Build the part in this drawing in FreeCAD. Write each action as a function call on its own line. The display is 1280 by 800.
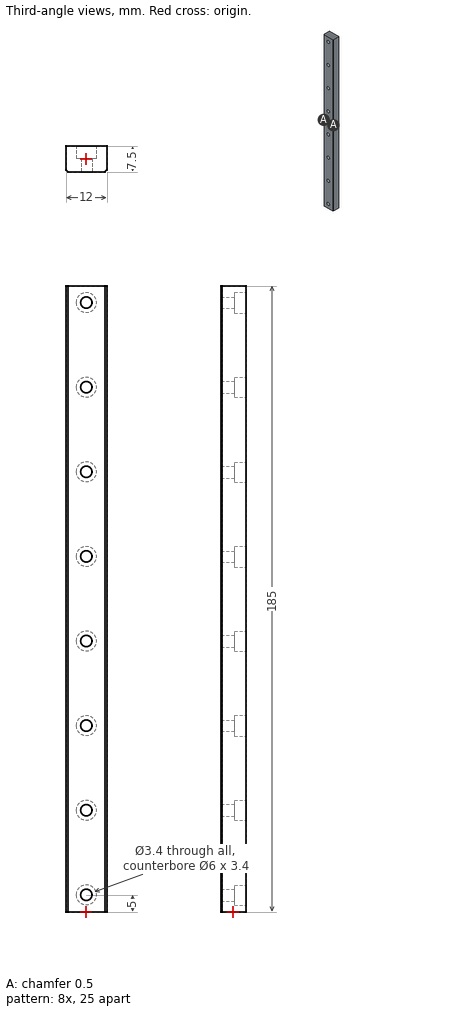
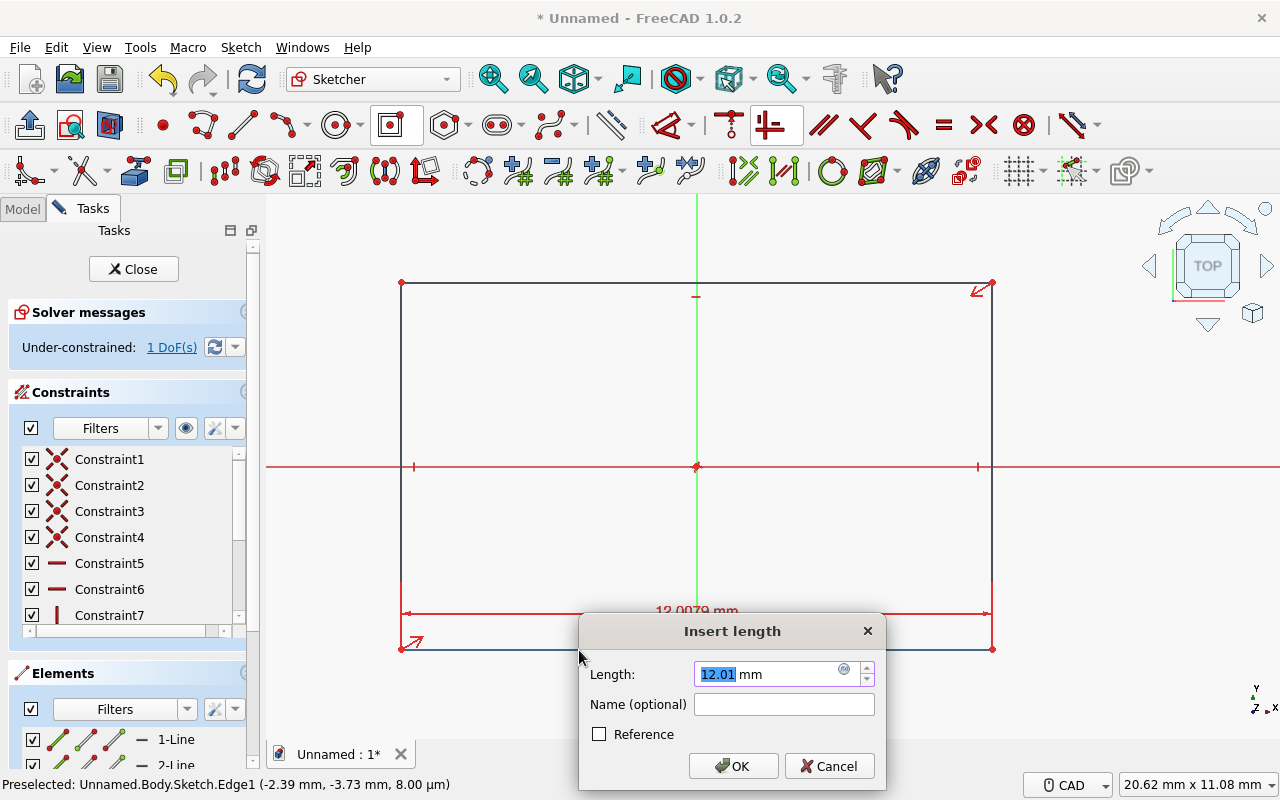
text(12)
key(Return)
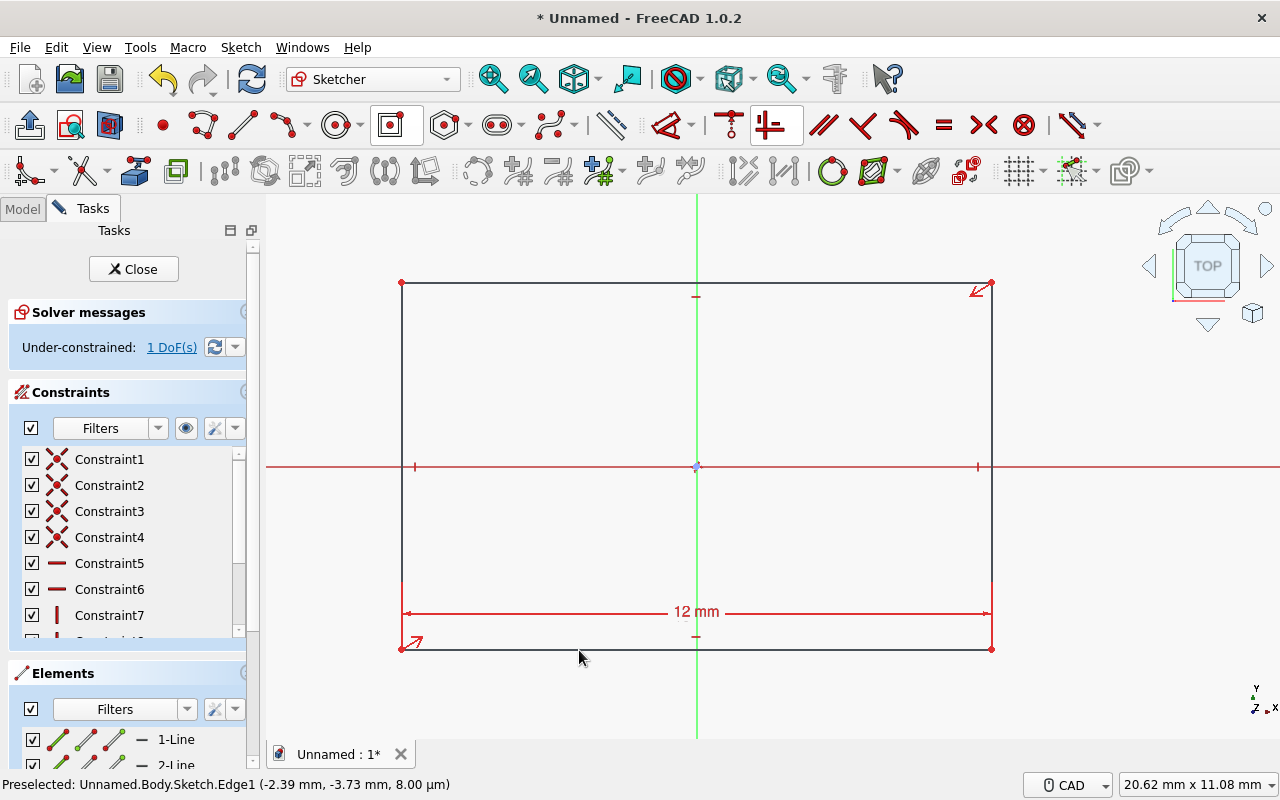
click(992, 540)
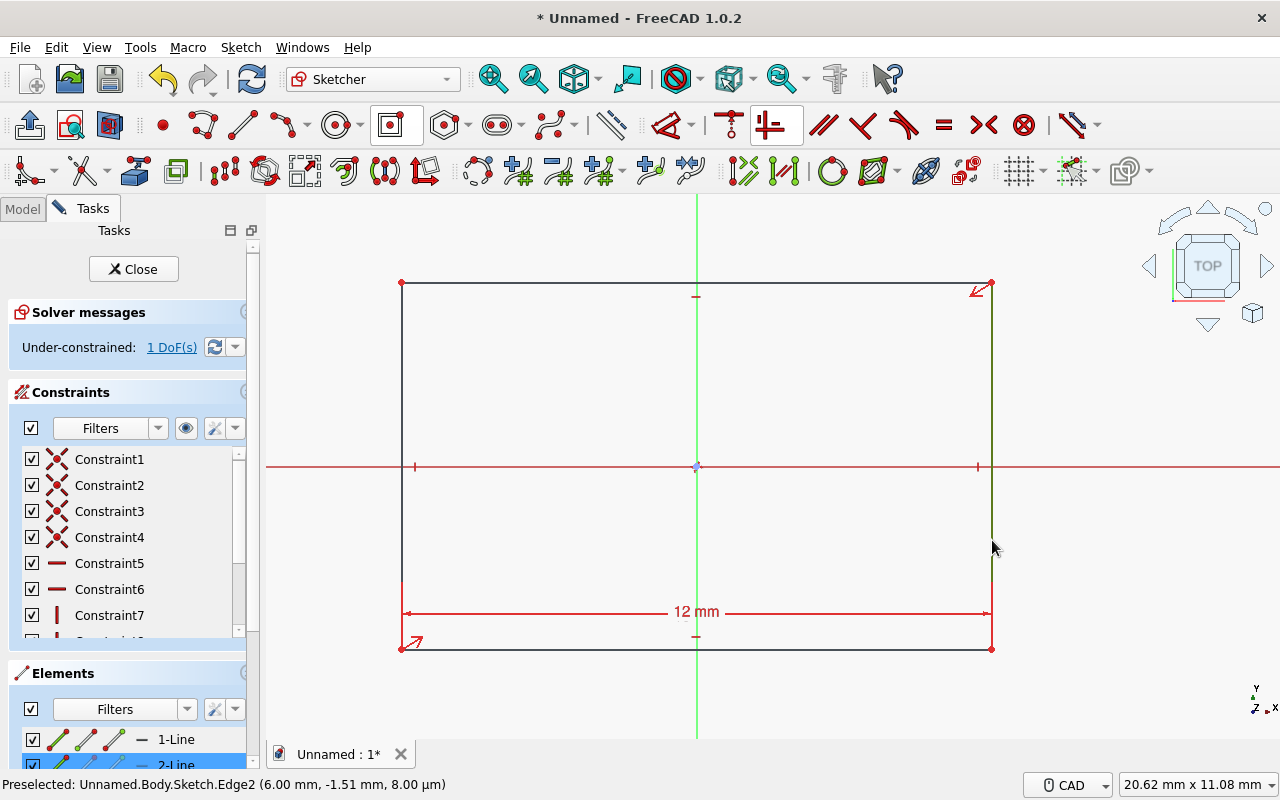
click(694, 126)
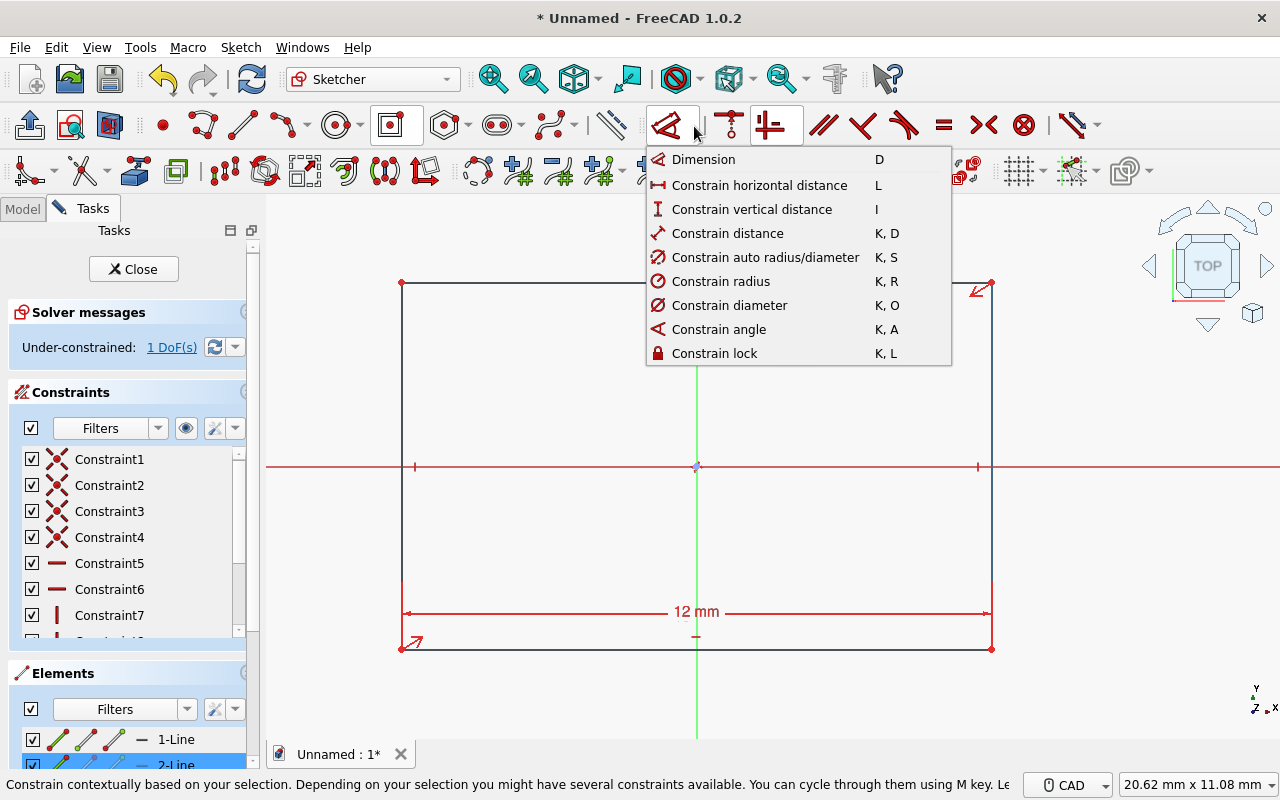
click(799, 209)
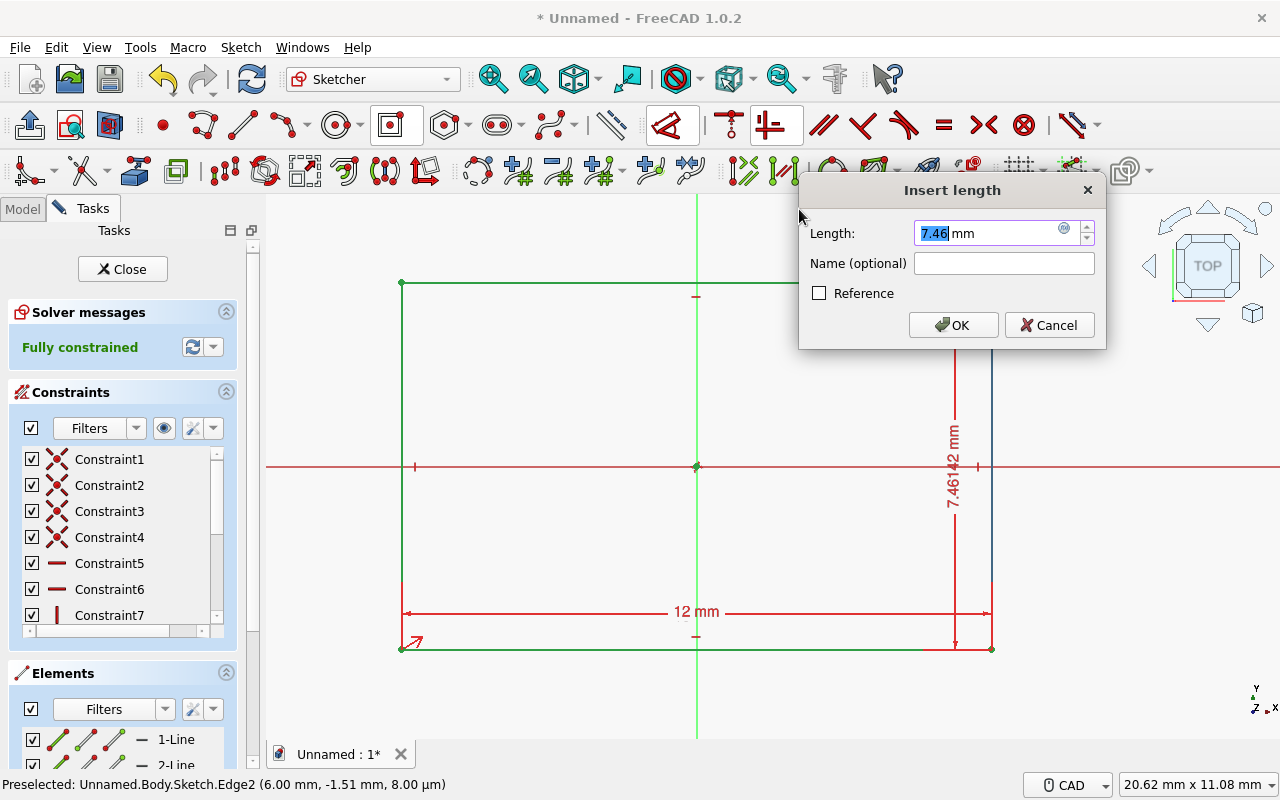
text(7.5)
key(Return)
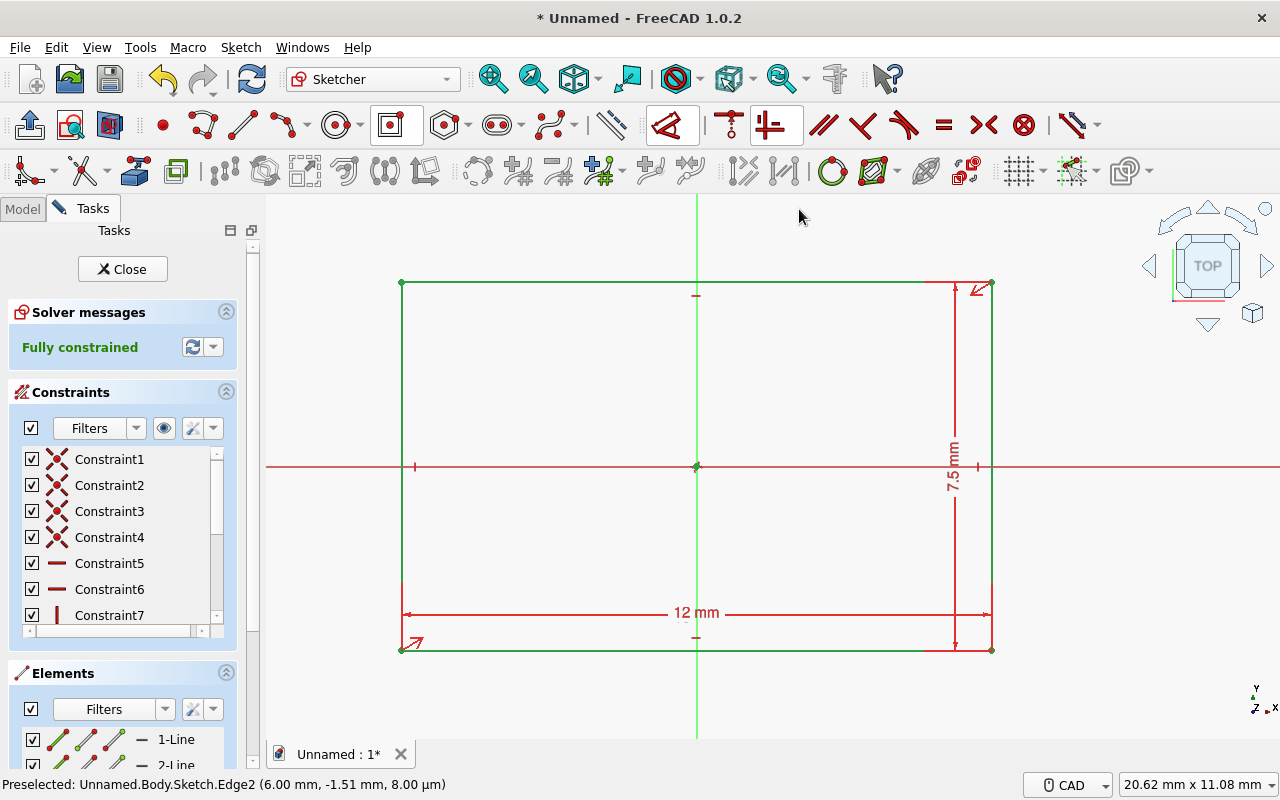
click(123, 269)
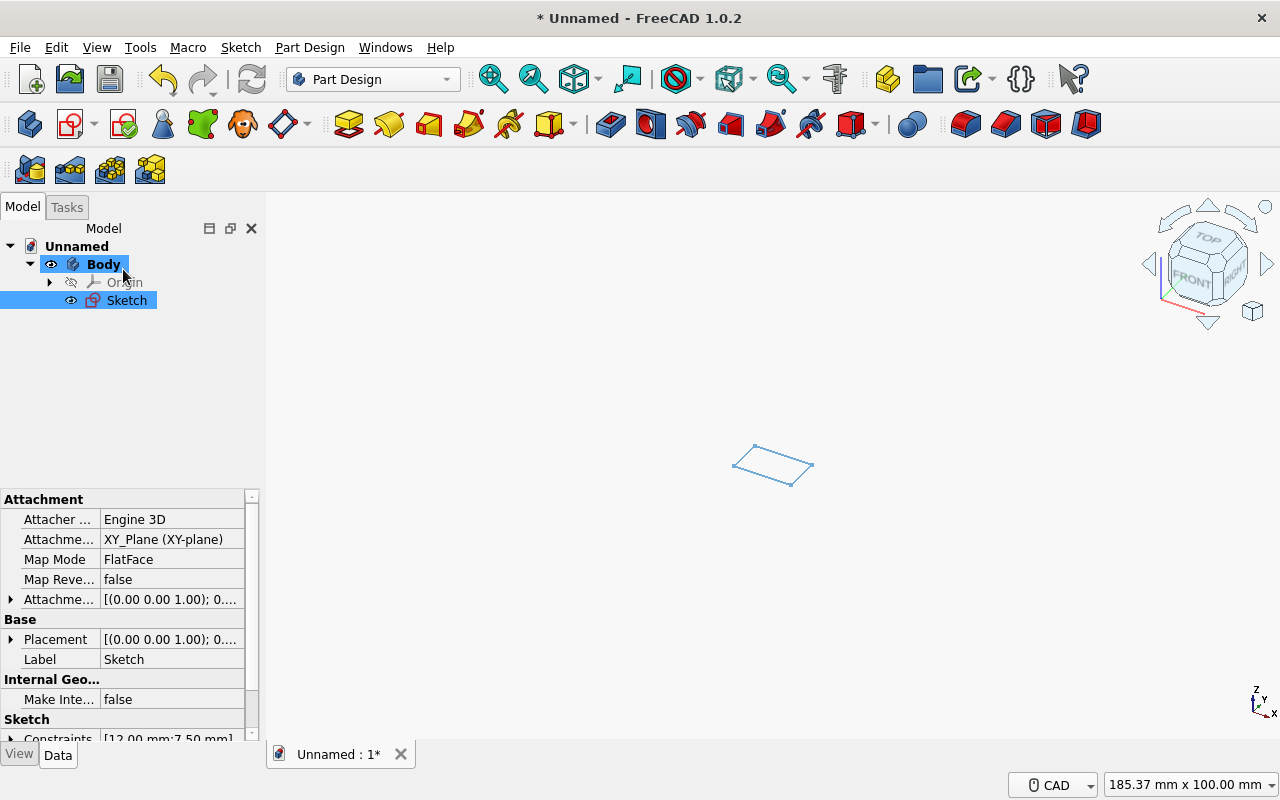
click(350, 124)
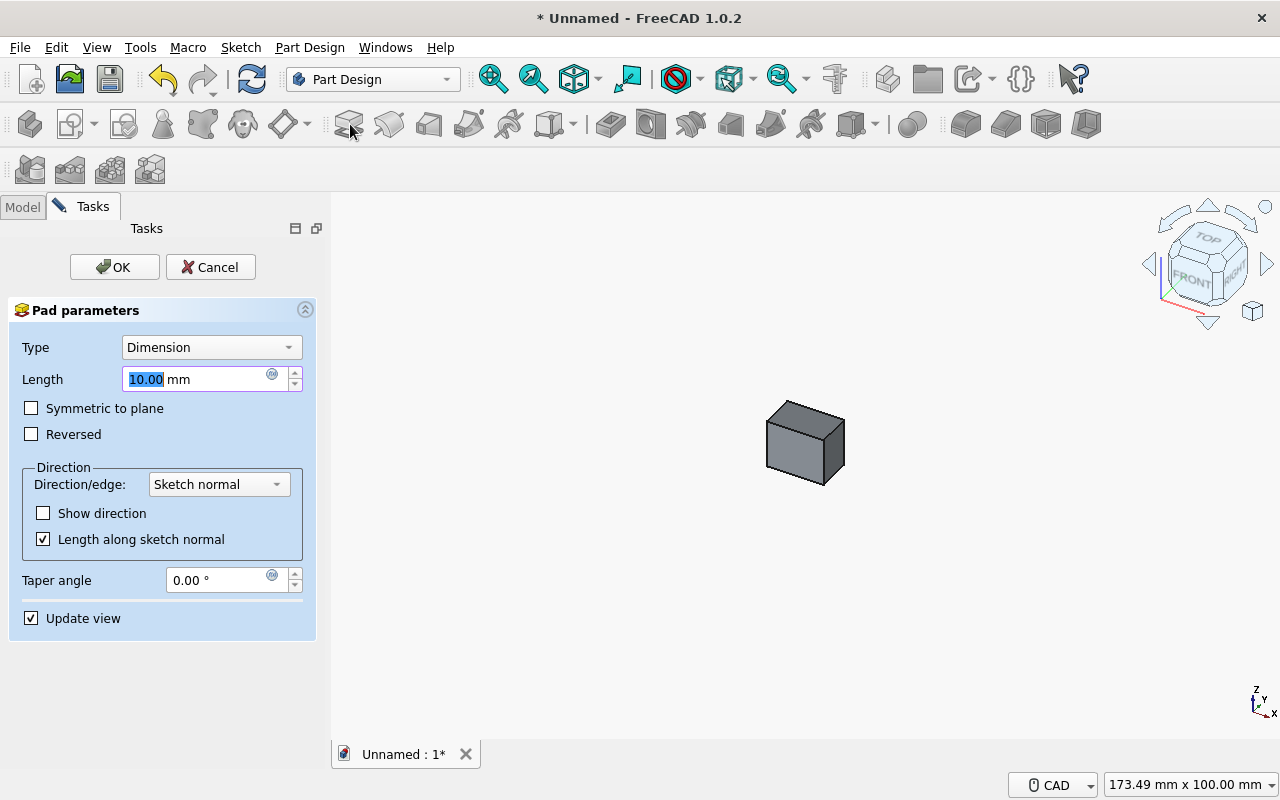
text(185)
key(Tab)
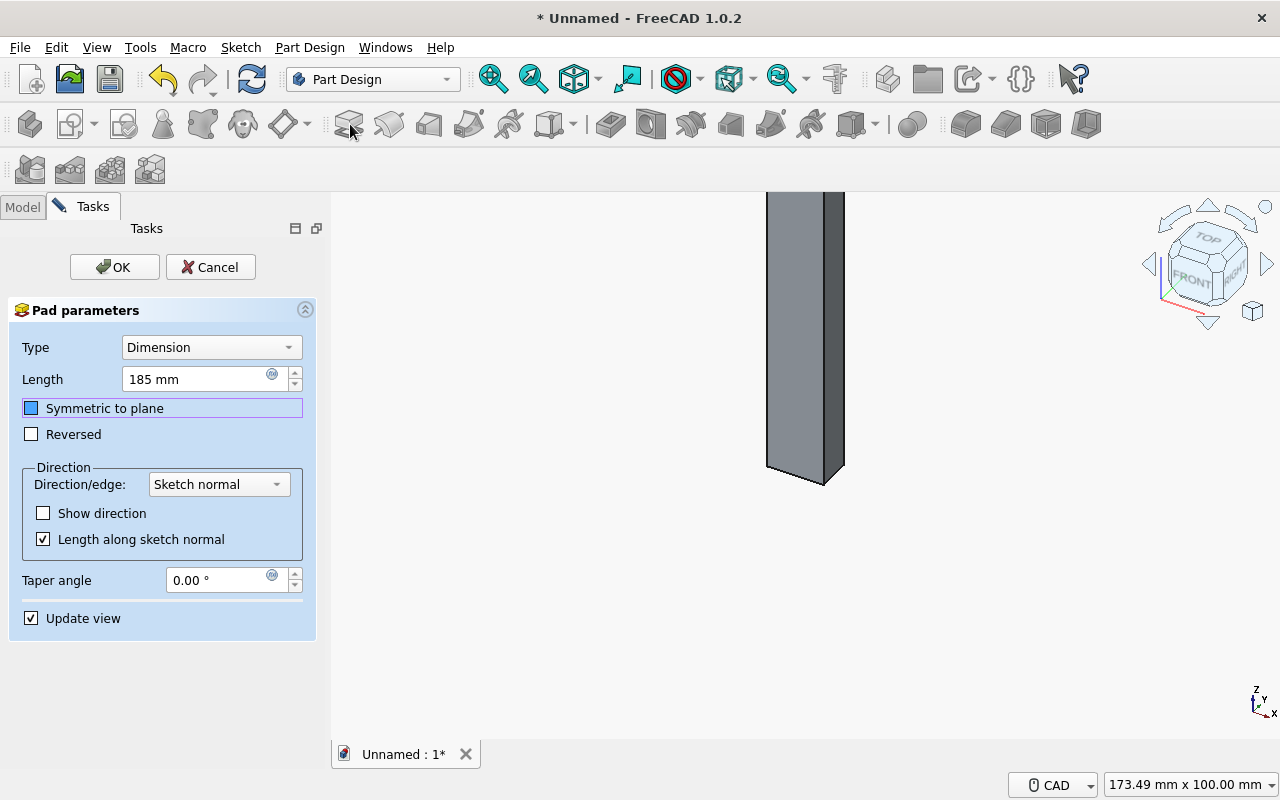
click(115, 267)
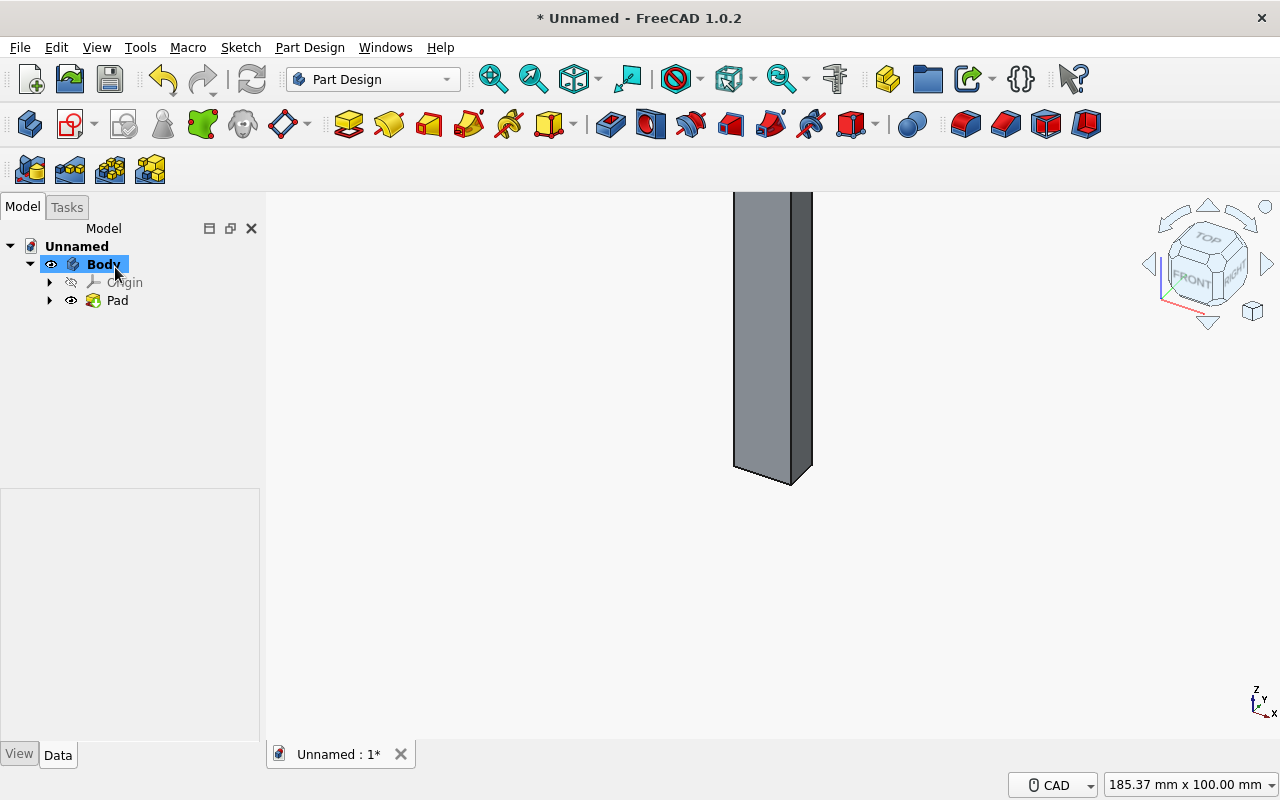
click(494, 80)